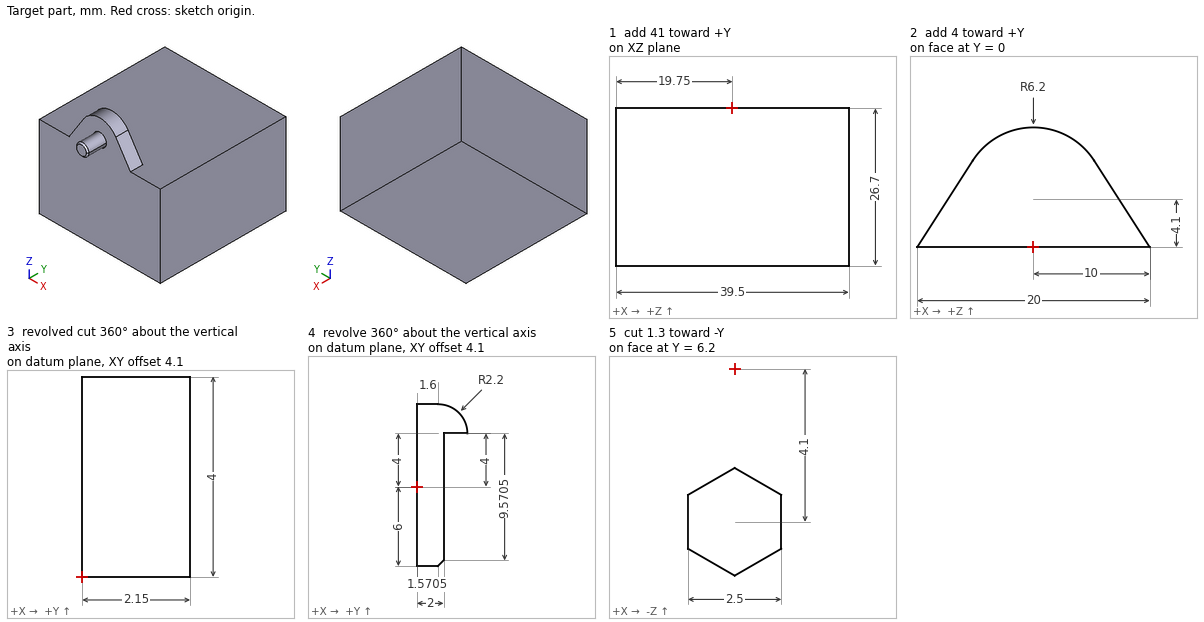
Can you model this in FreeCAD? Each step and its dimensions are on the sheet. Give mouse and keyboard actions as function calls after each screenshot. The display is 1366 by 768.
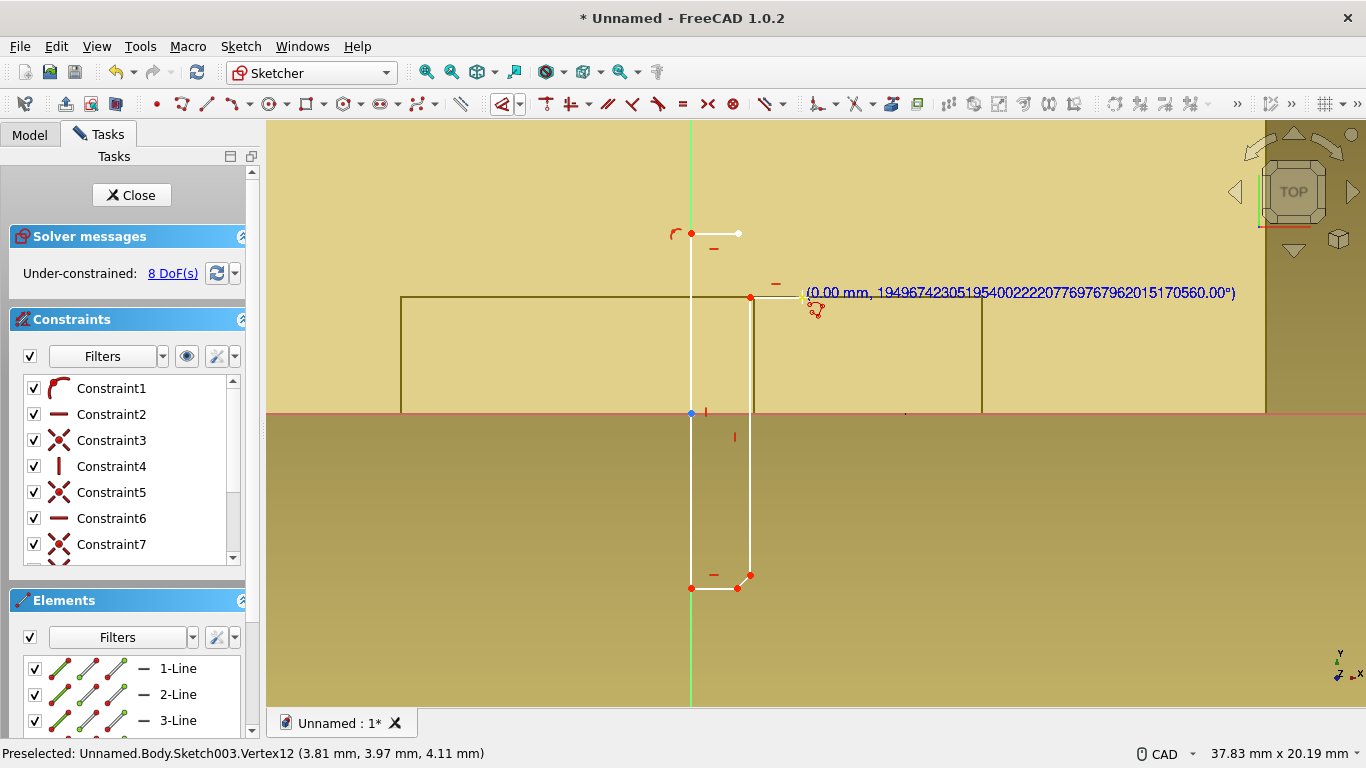
click(232, 104)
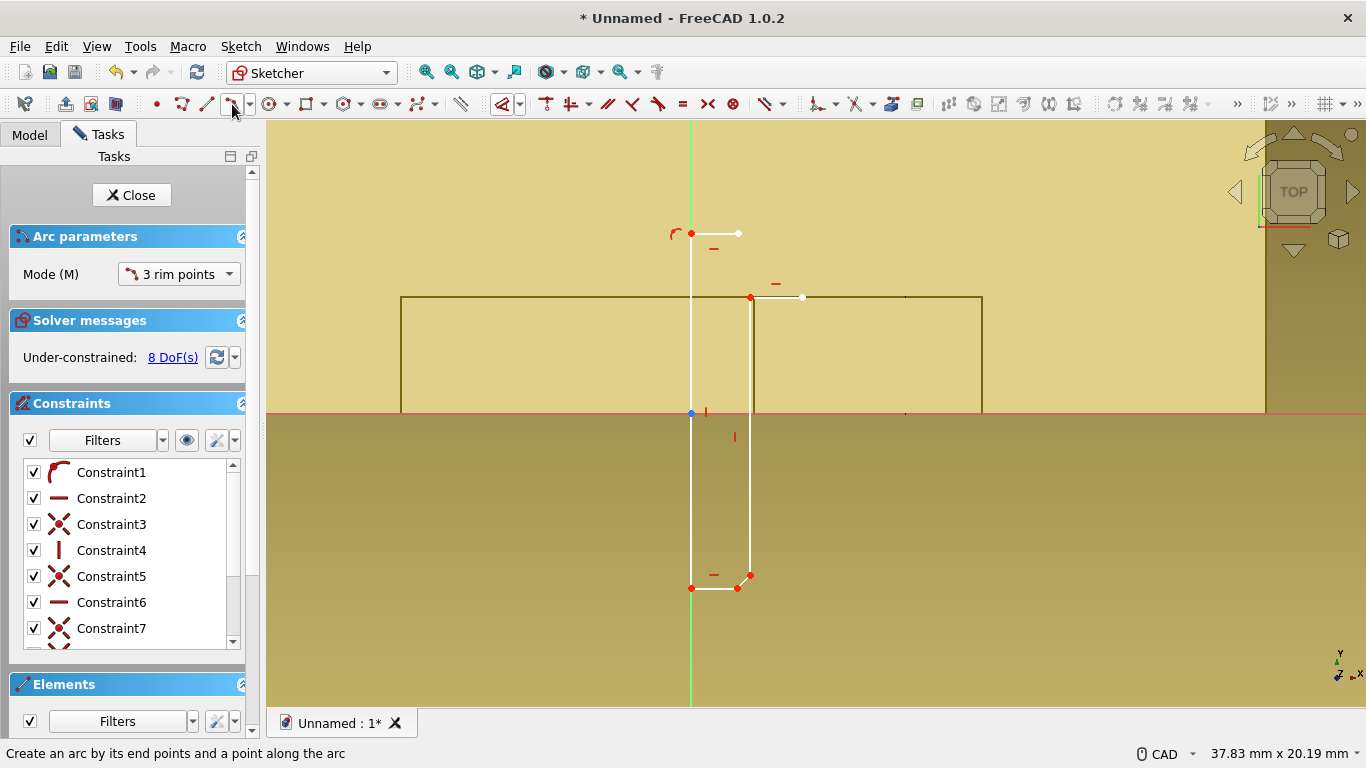
click(802, 298)
click(738, 234)
click(783, 252)
key(Escape)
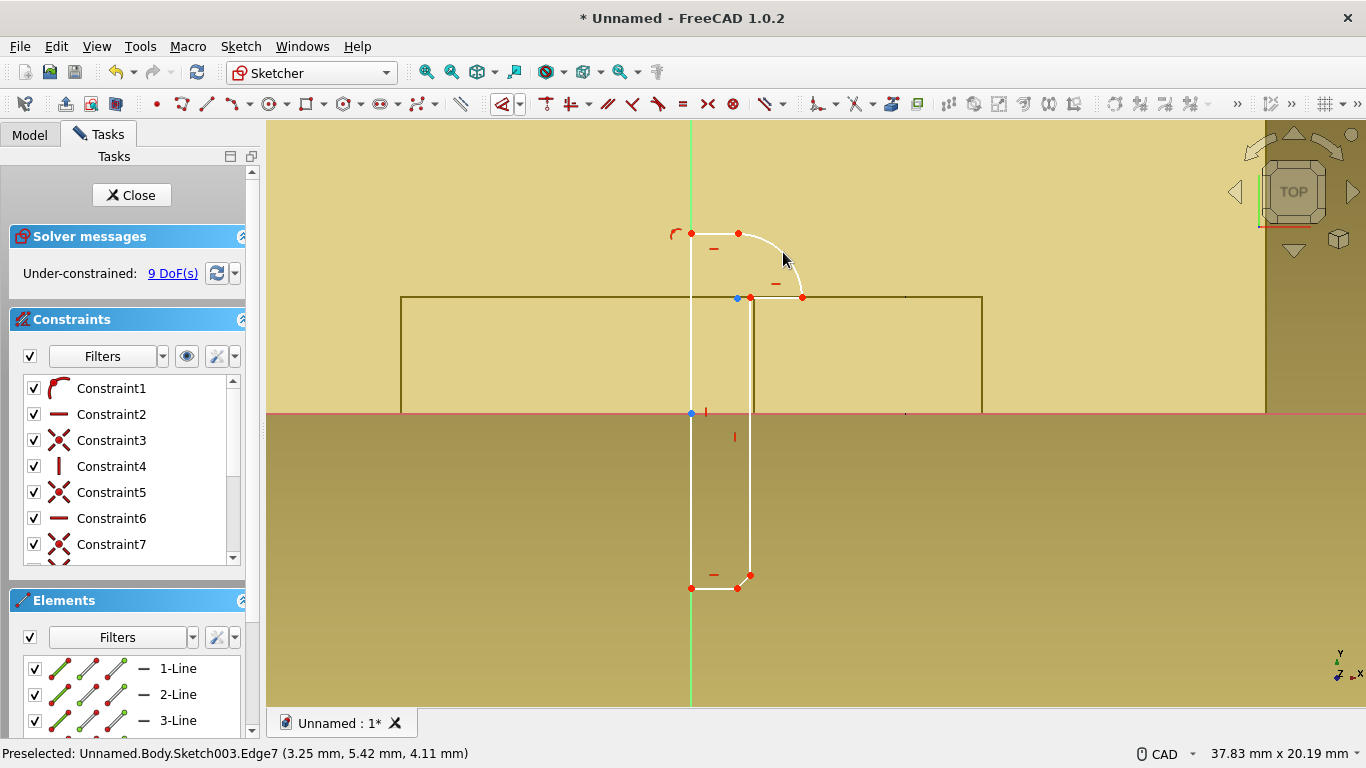
click(724, 234)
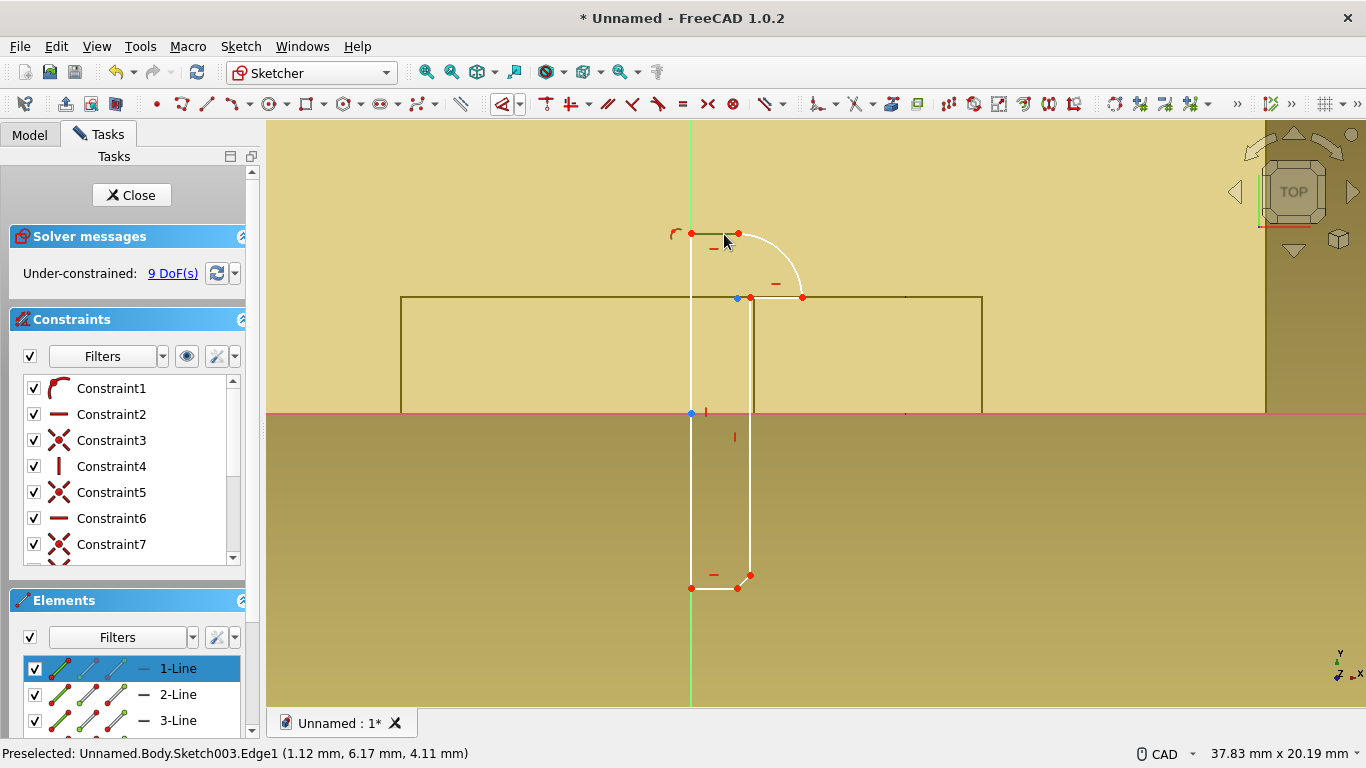
click(795, 269)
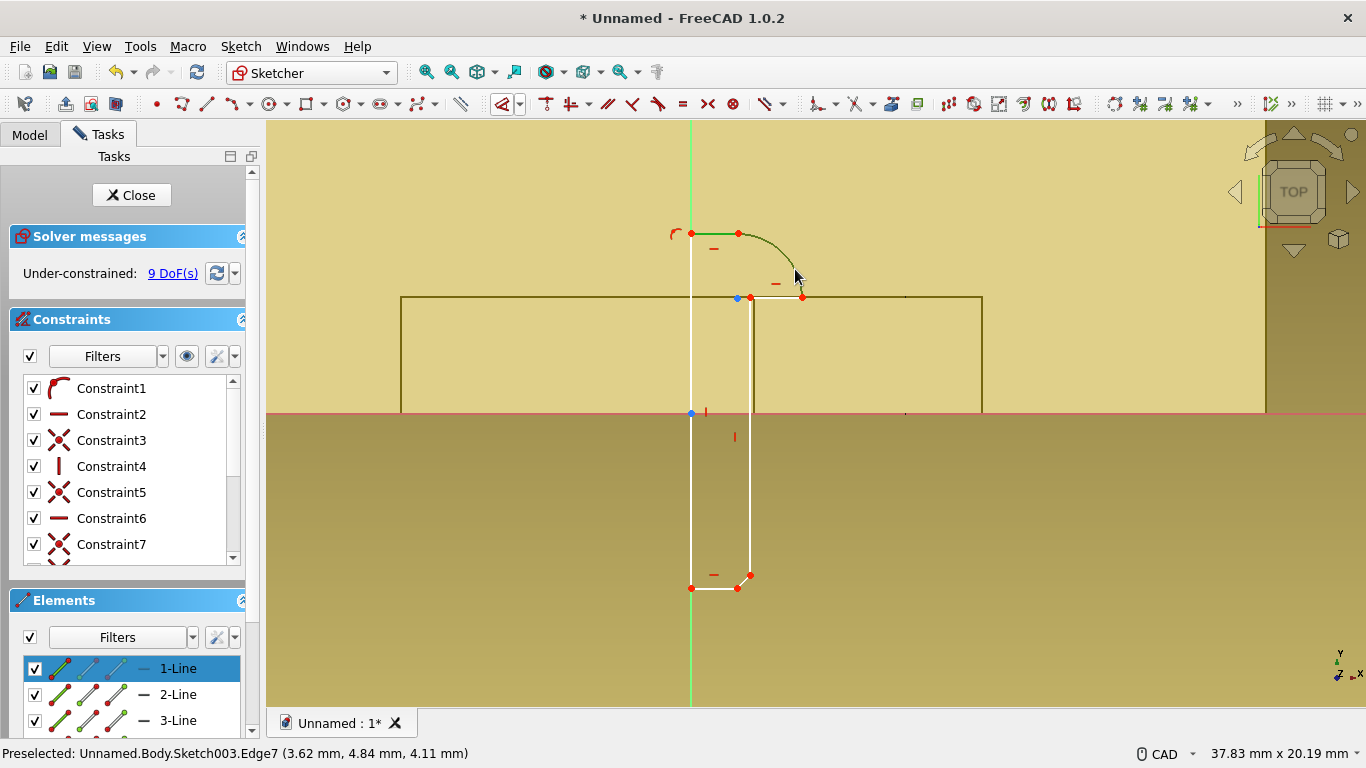
key(t)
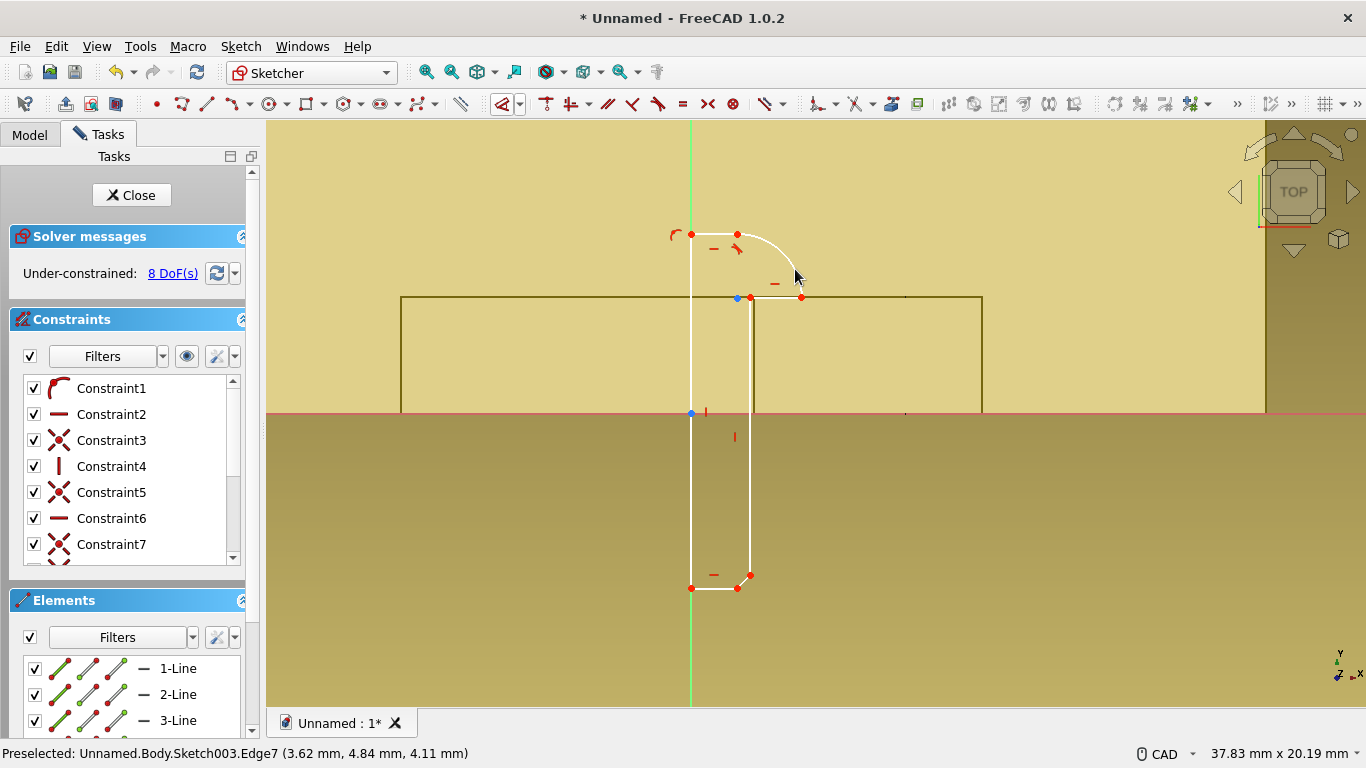
click(795, 269)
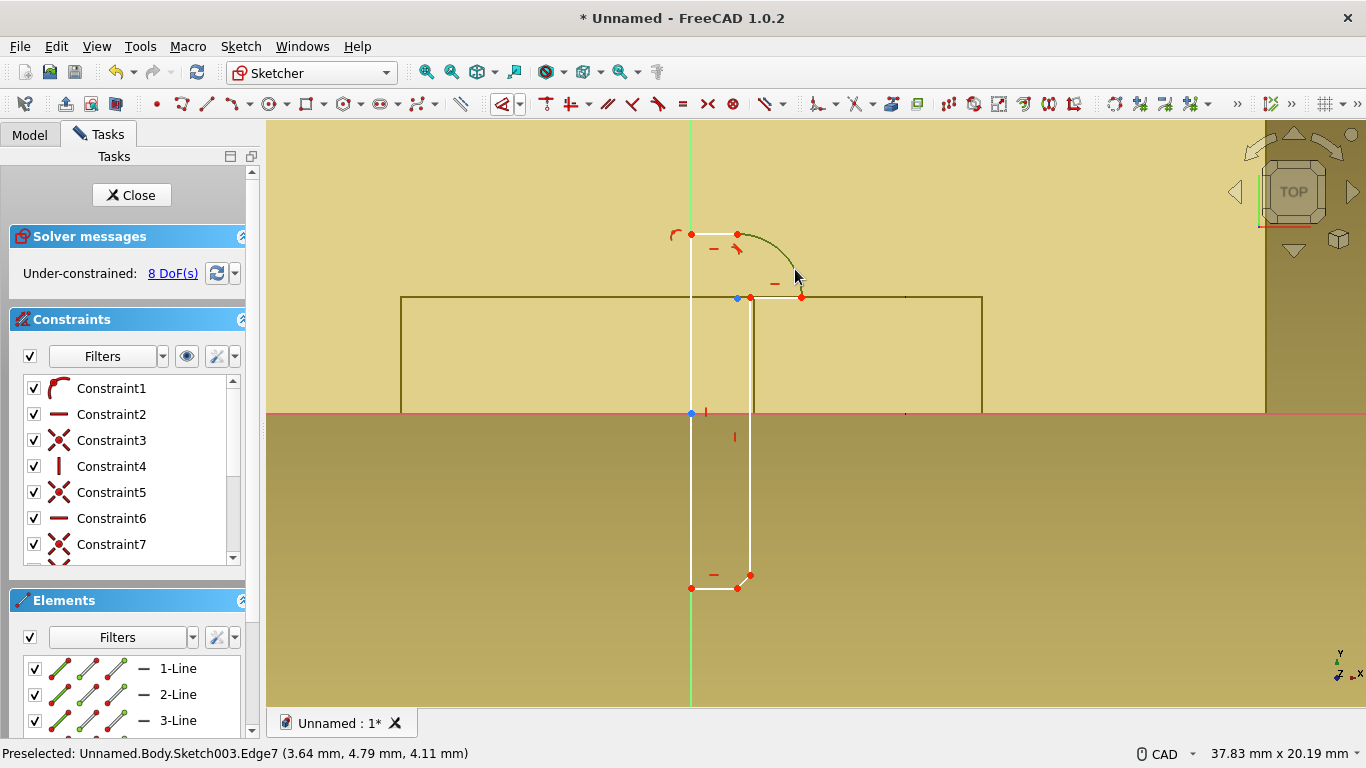
key(k)
key(r)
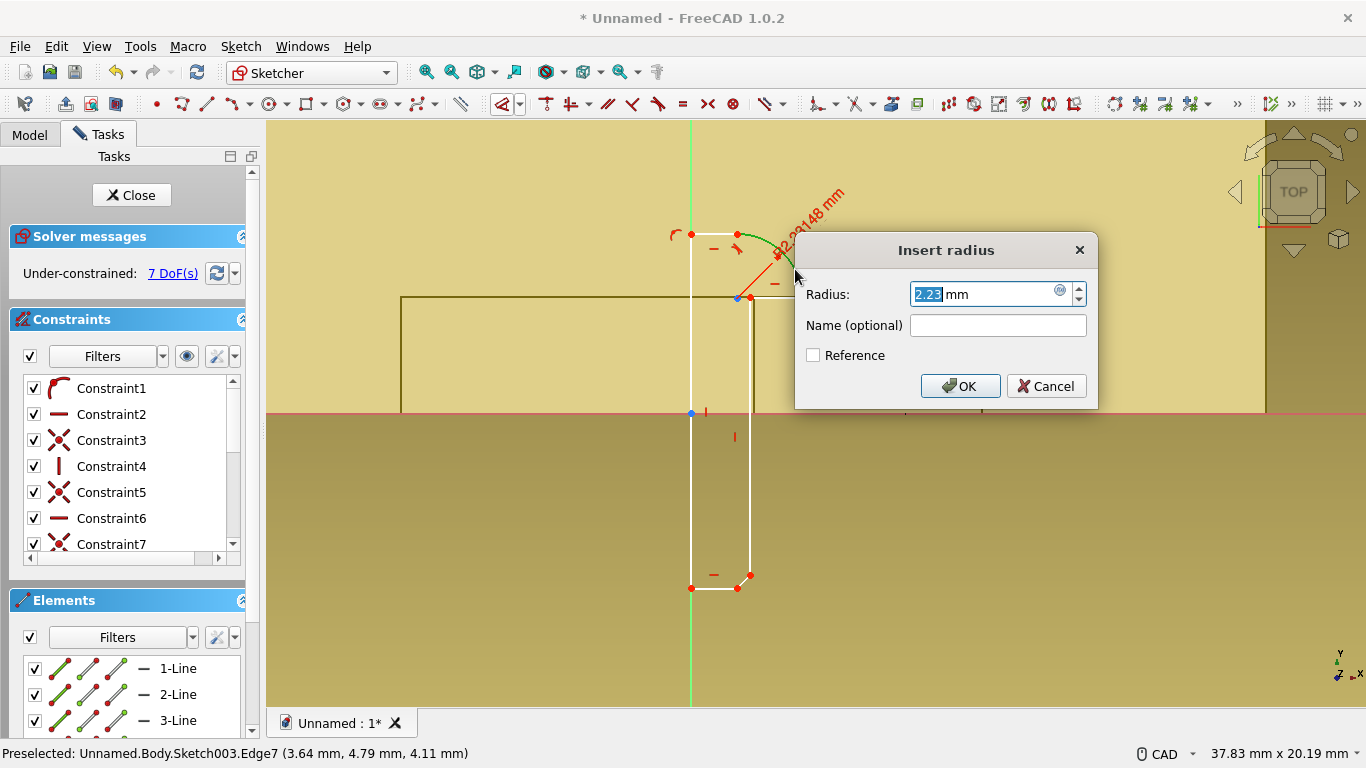
text(2.2)
key(Return)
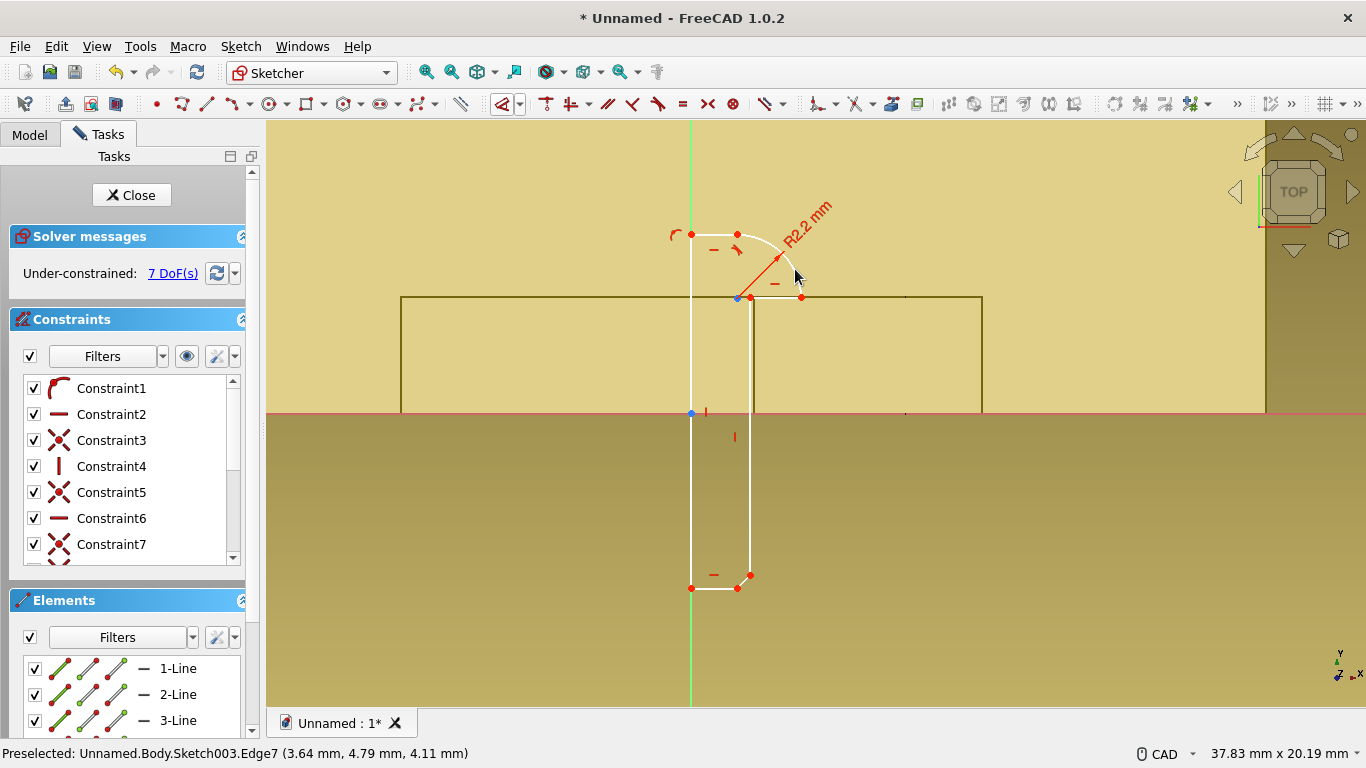
click(691, 589)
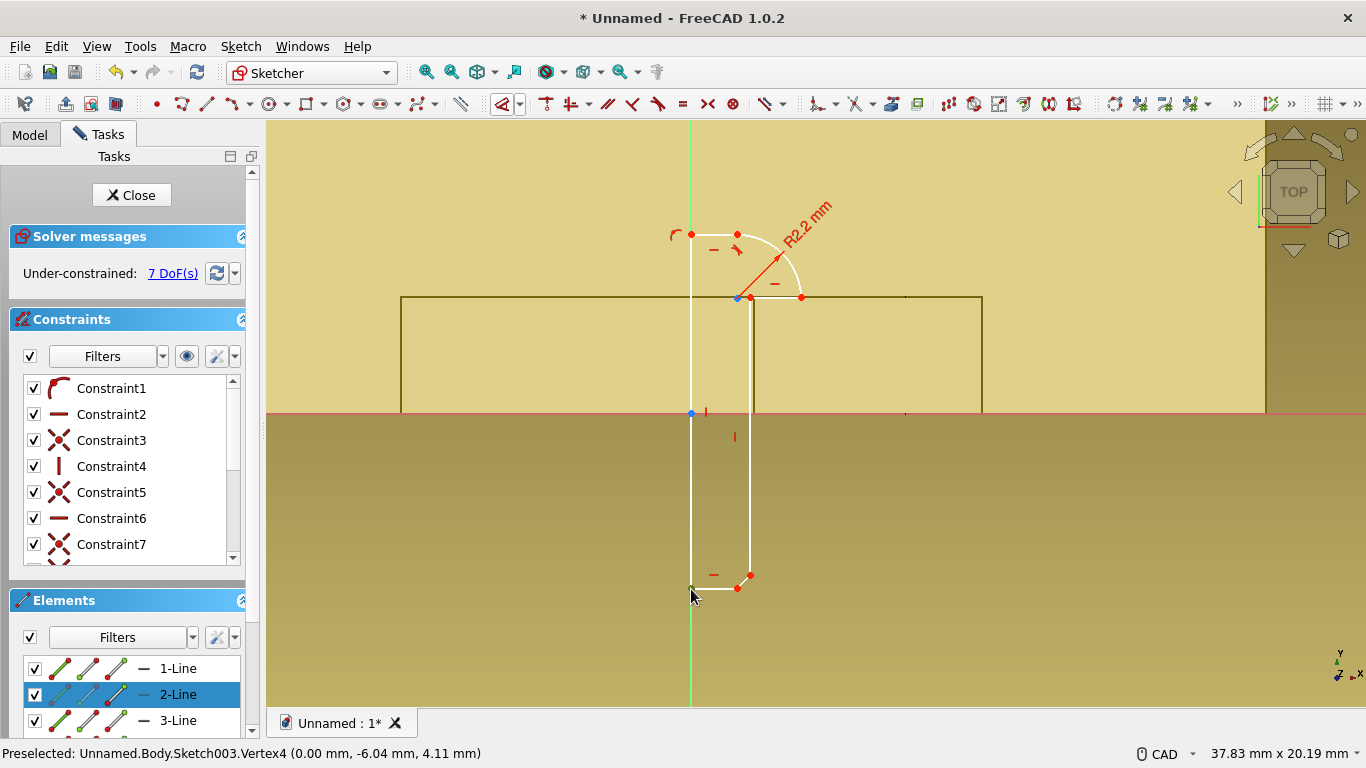
click(520, 104)